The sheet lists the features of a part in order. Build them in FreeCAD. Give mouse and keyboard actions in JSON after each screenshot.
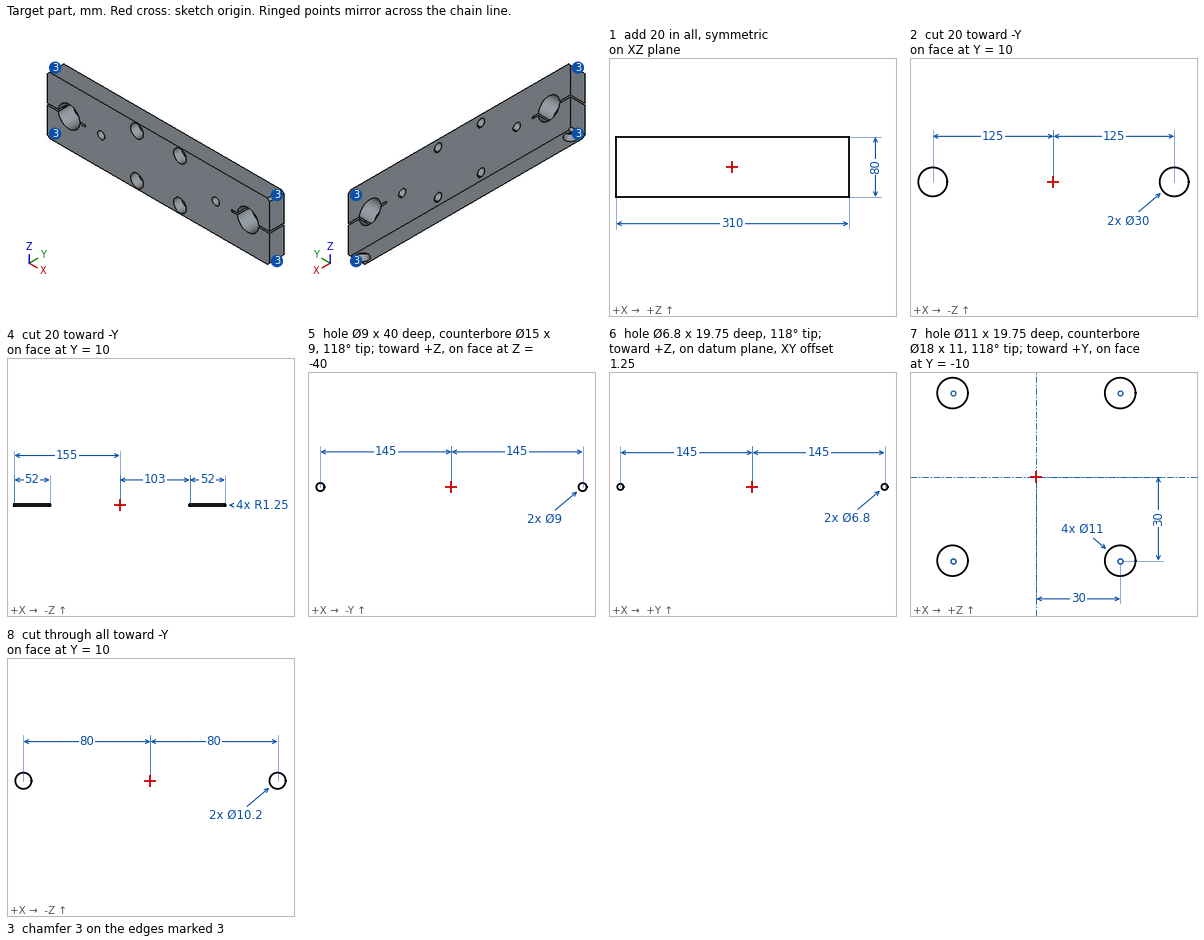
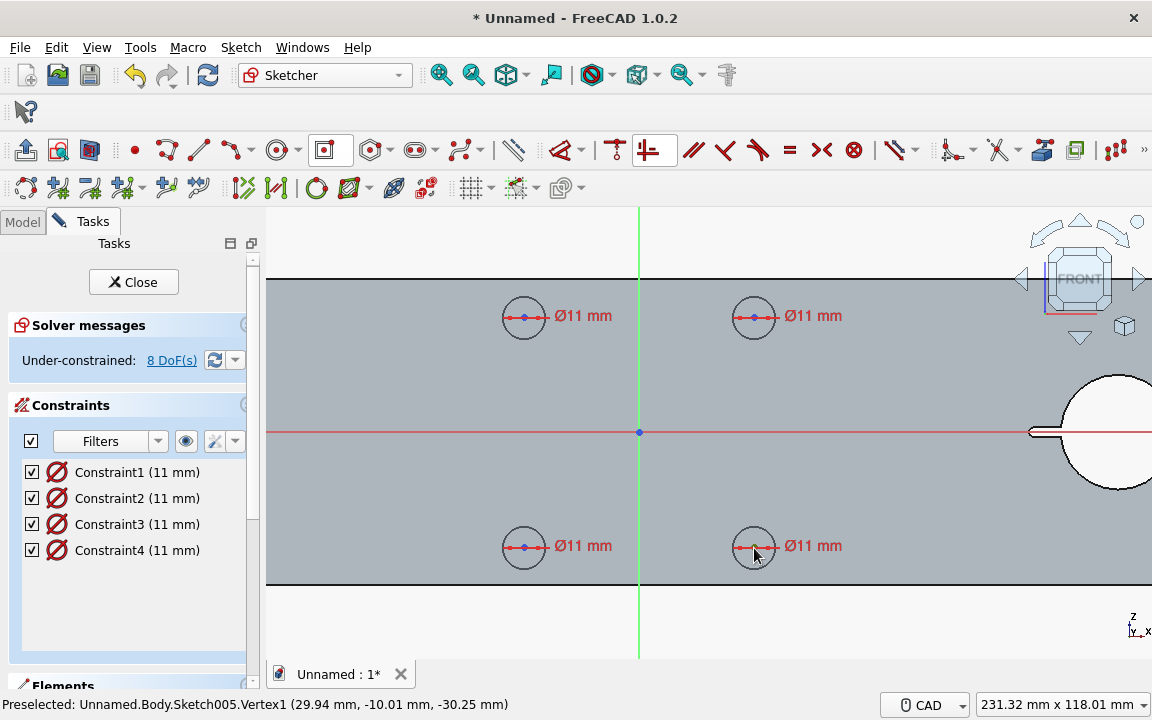
{"action": "left_click", "coordinate": [524, 548]}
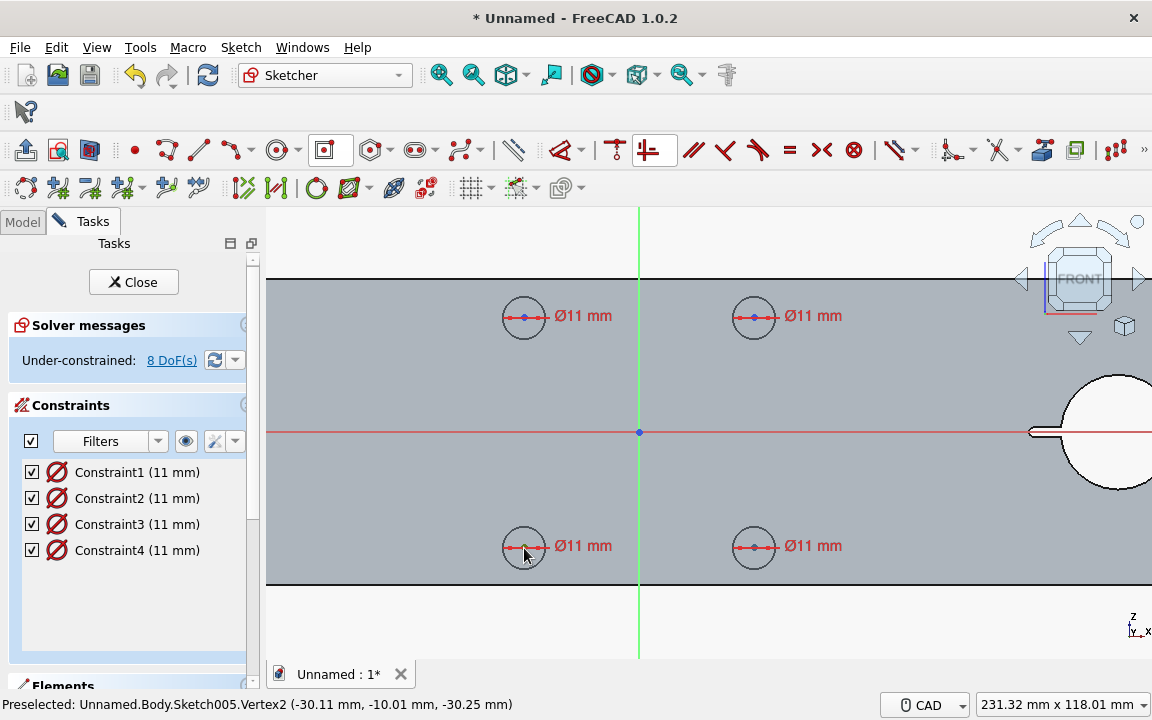
{"action": "left_click", "coordinate": [639, 603]}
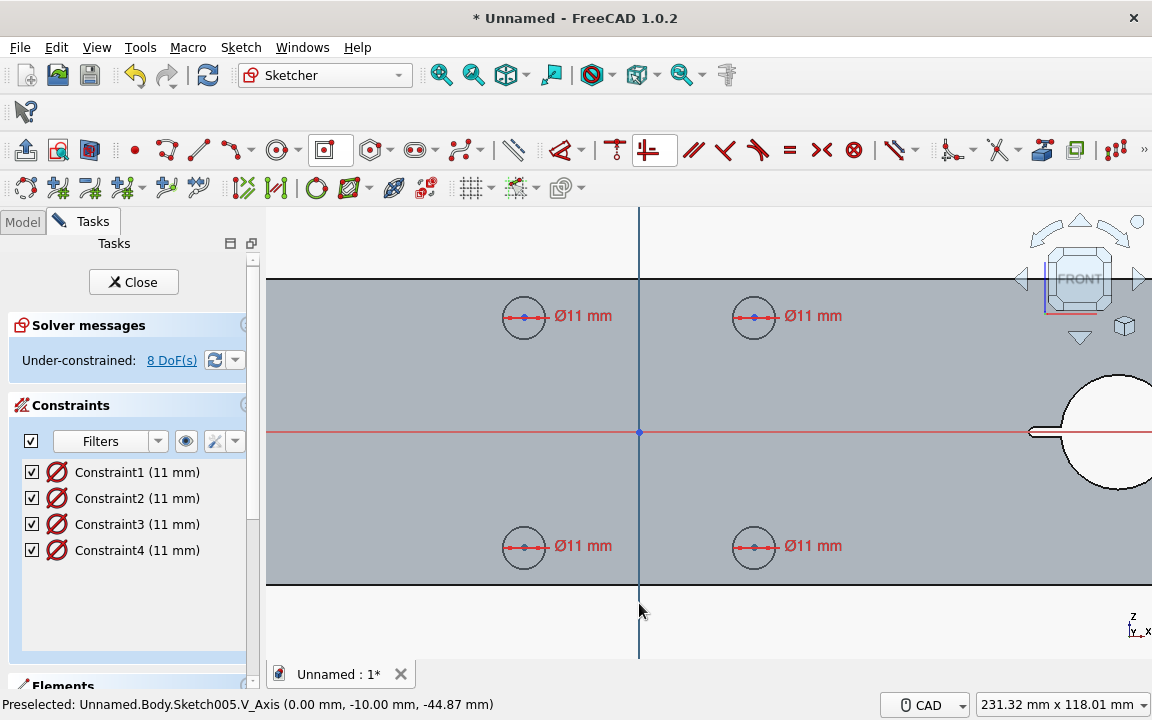
{"action": "left_click", "coordinate": [822, 150]}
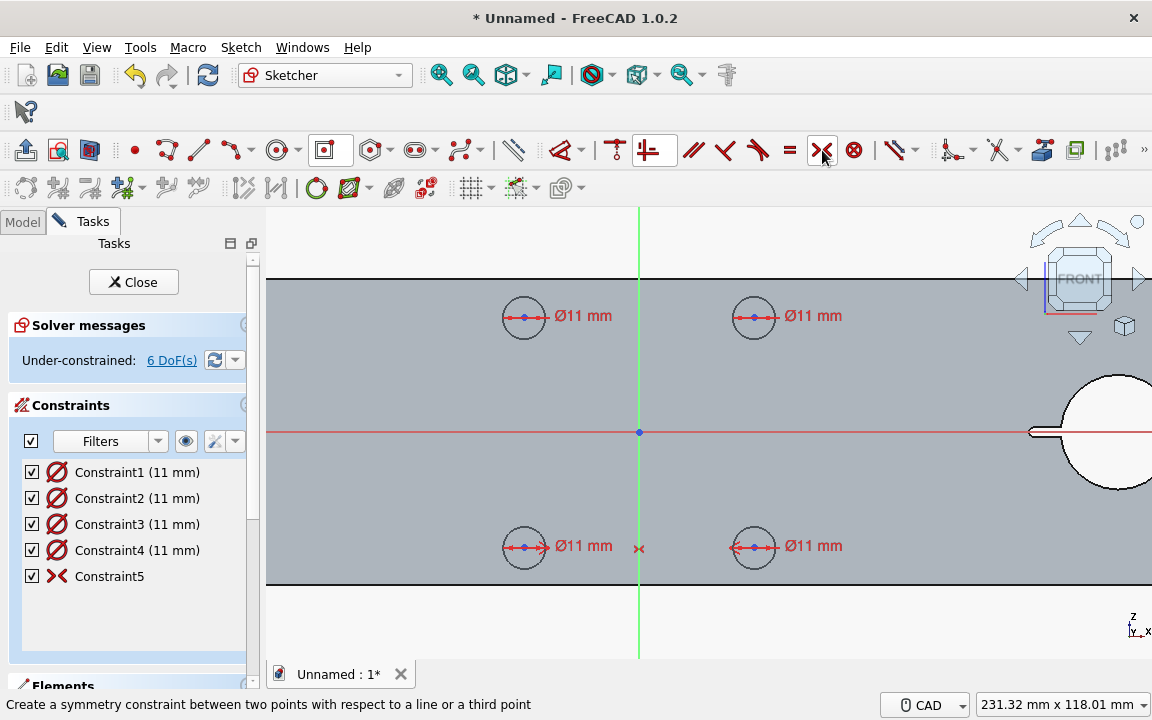
{"action": "left_click", "coordinate": [524, 548]}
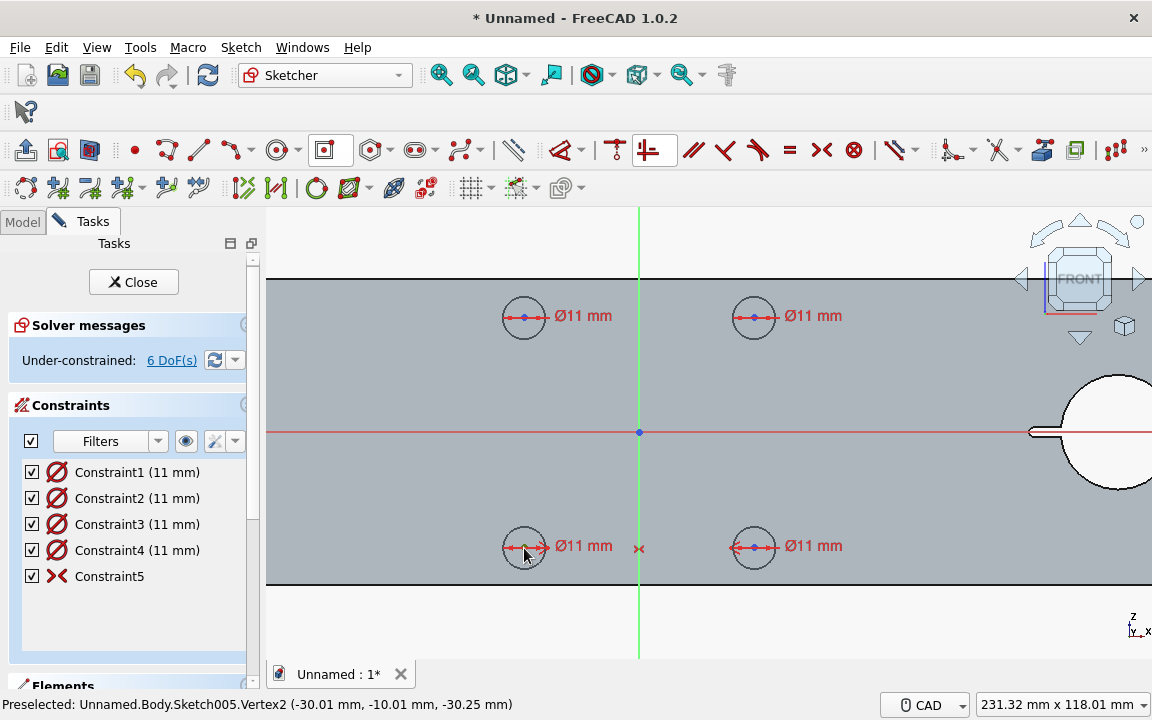
{"action": "left_click", "coordinate": [524, 318]}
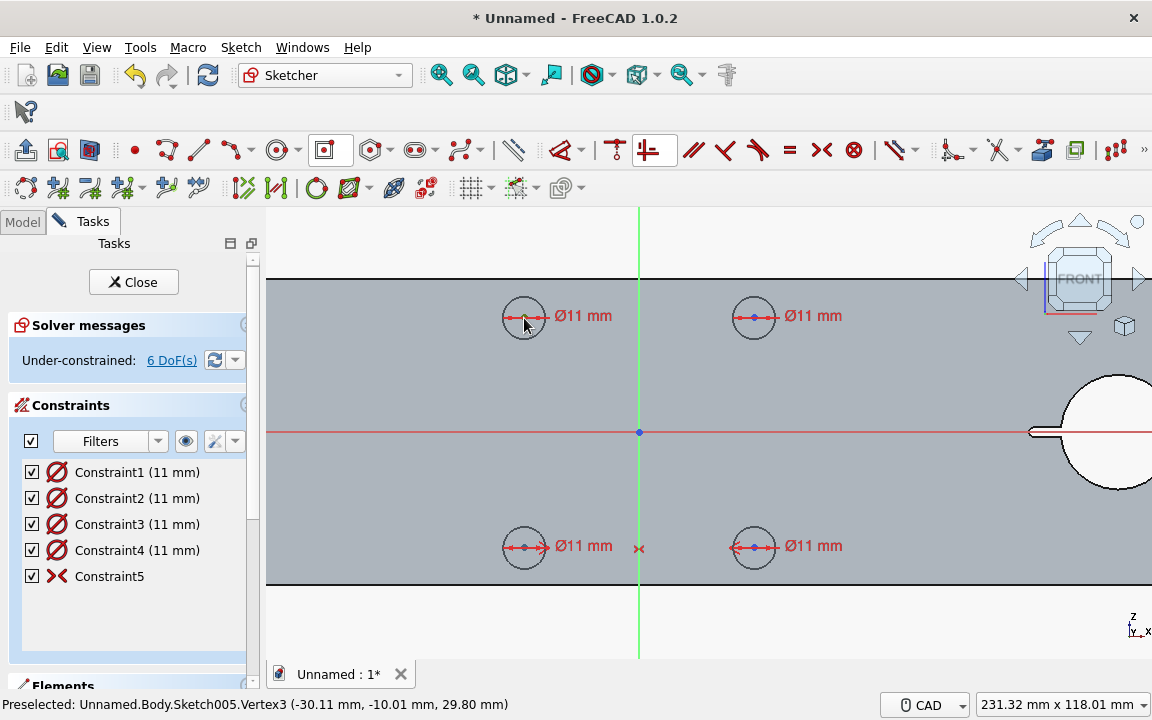
{"action": "left_click", "coordinate": [343, 432]}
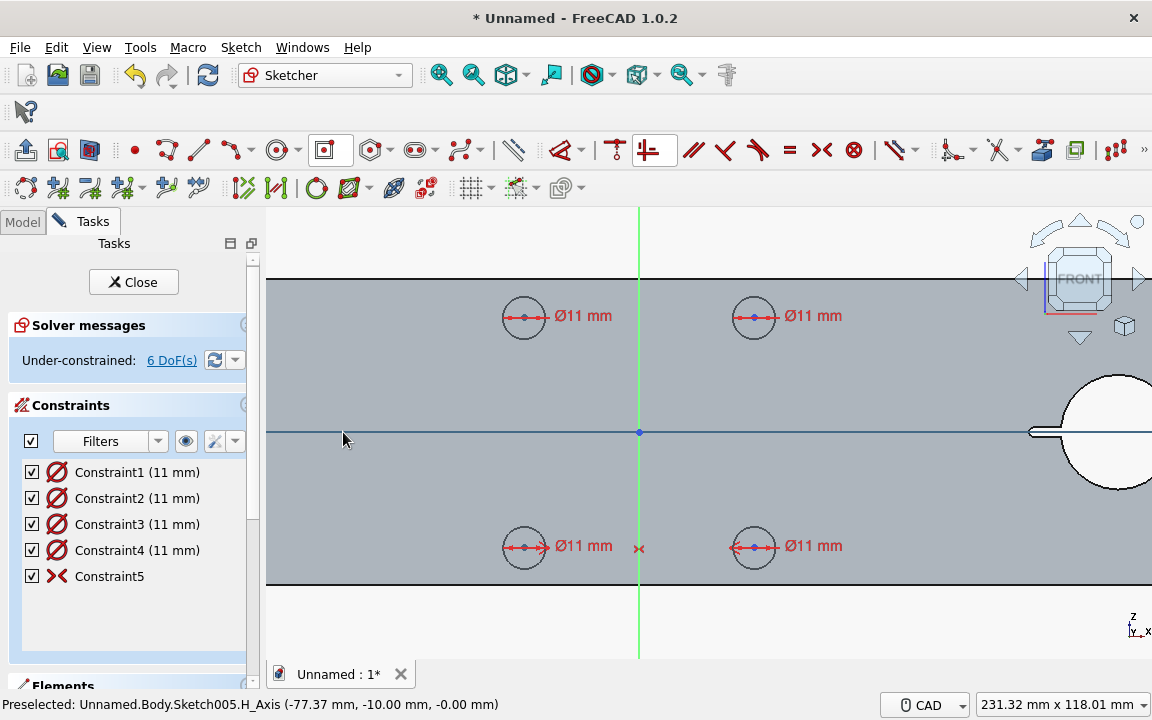
{"action": "left_click", "coordinate": [822, 150]}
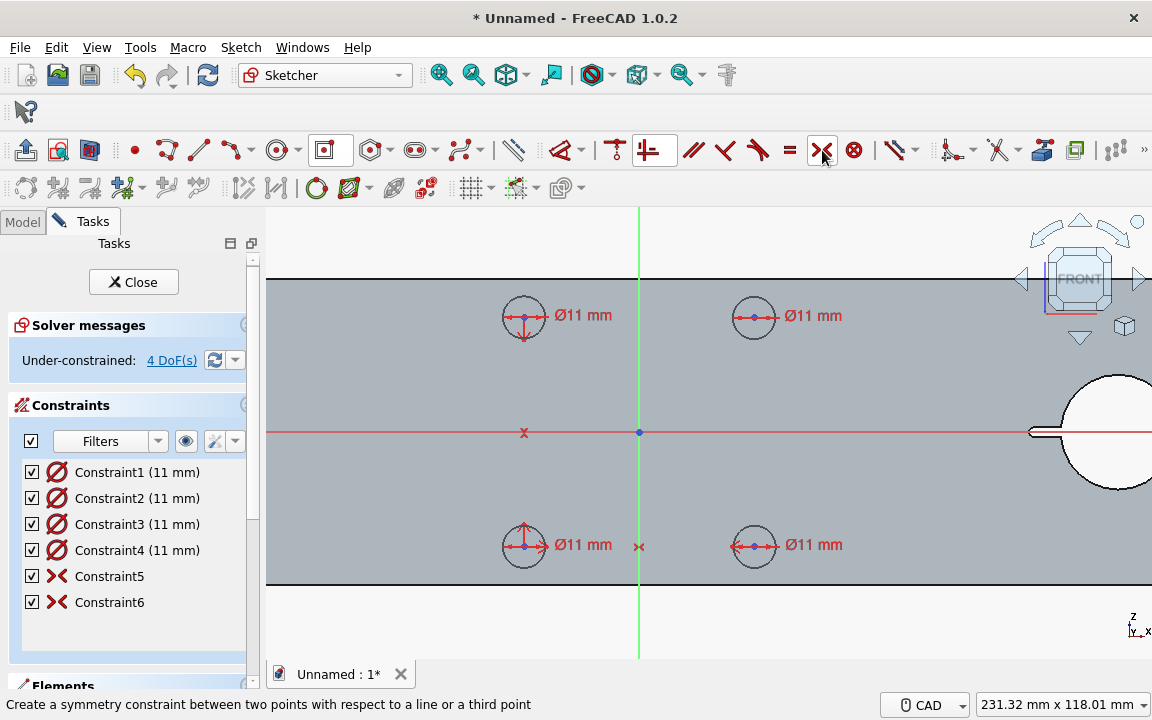
{"action": "left_click", "coordinate": [755, 547]}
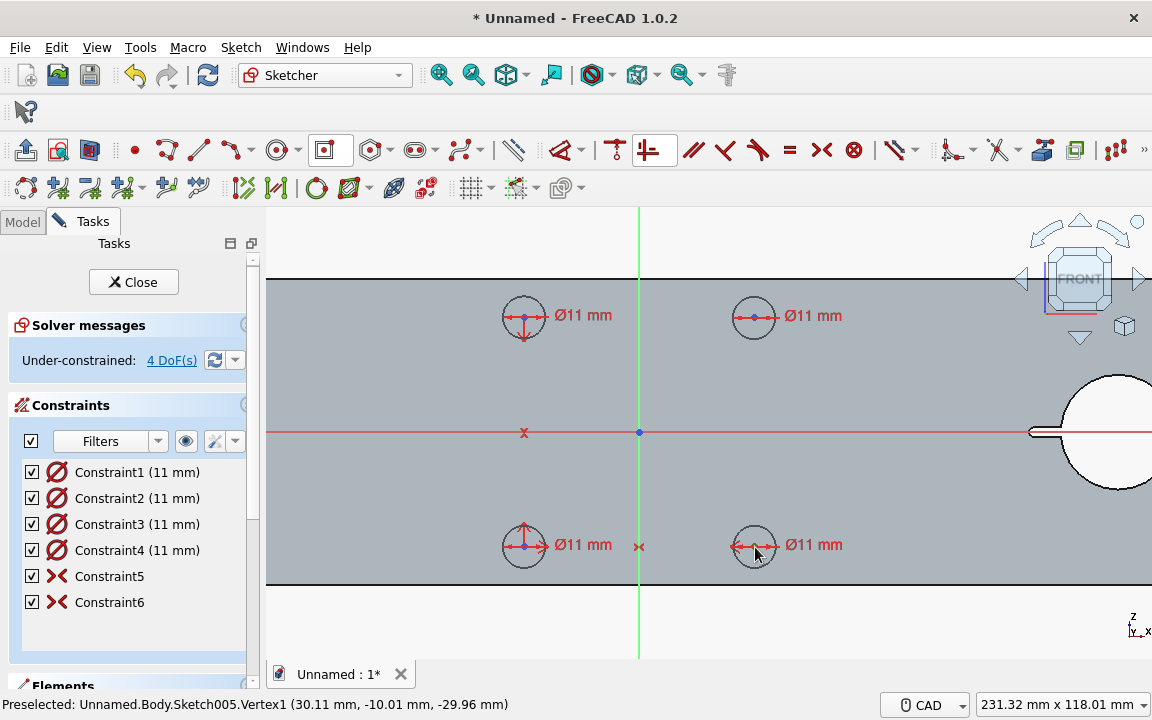
{"action": "left_click", "coordinate": [754, 318]}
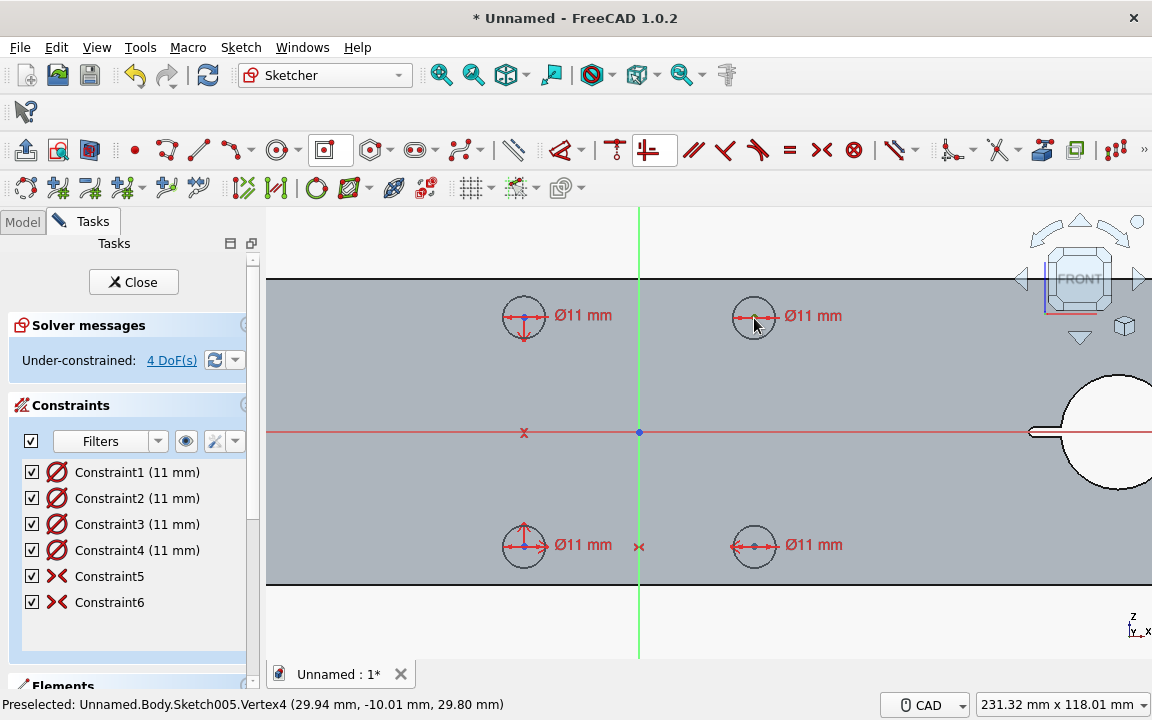
{"action": "left_click", "coordinate": [343, 432]}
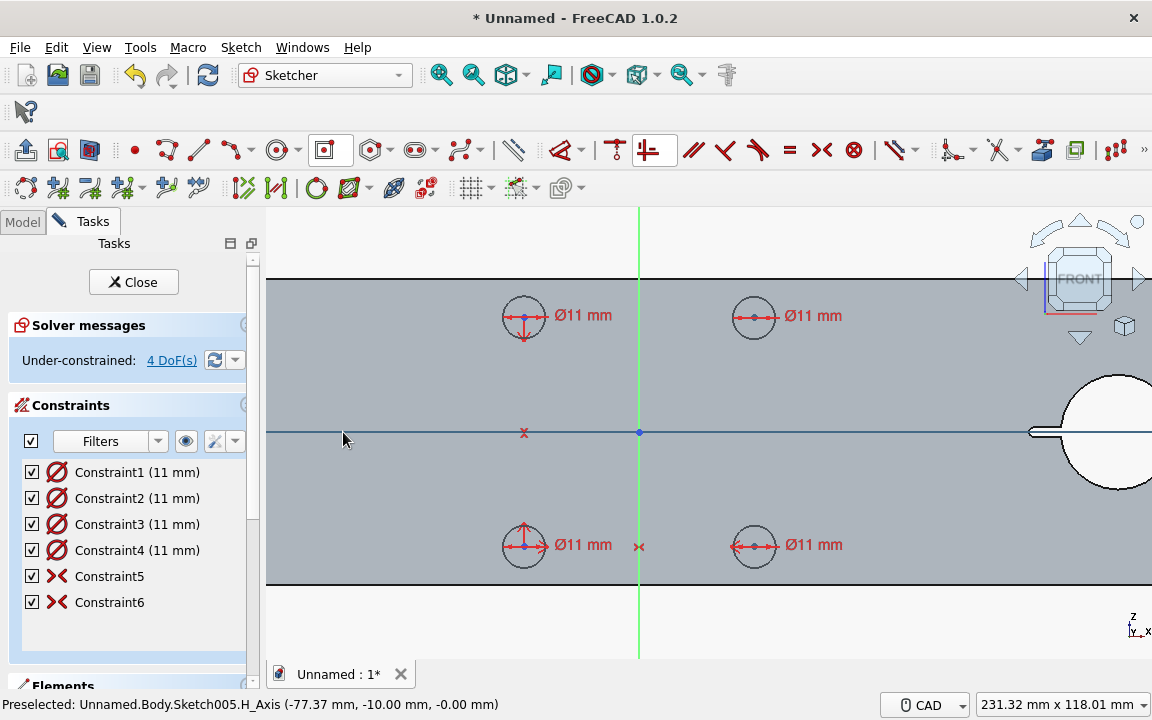
{"action": "left_click", "coordinate": [822, 150]}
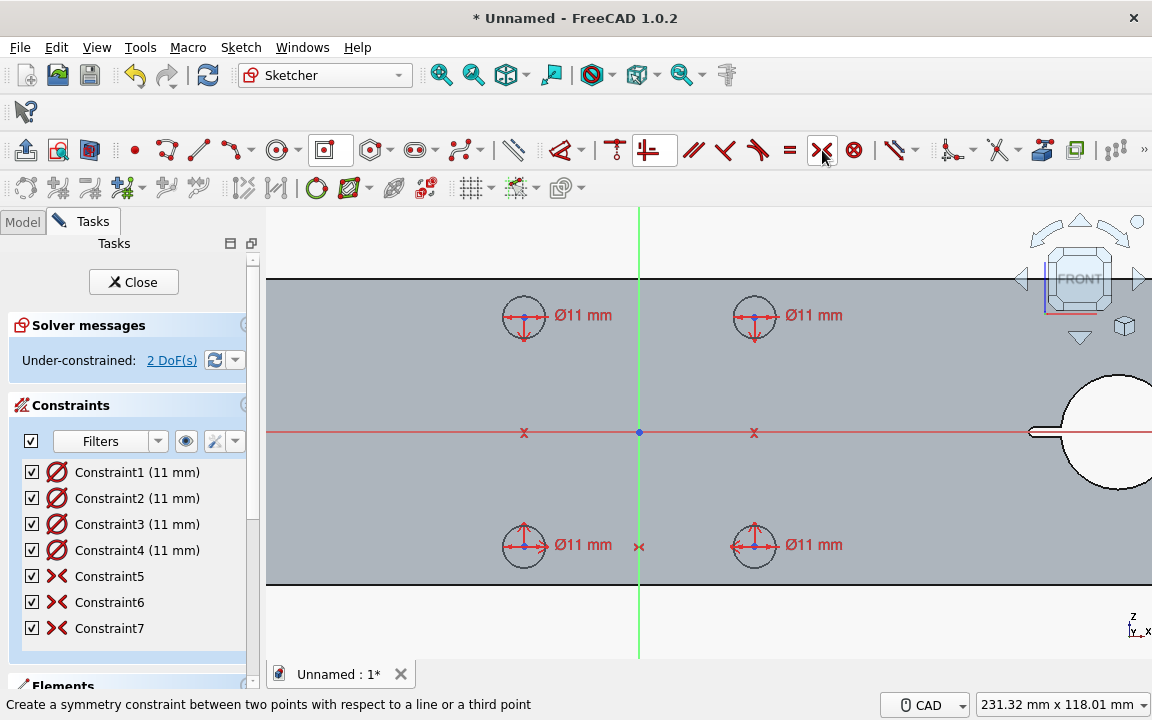
{"action": "left_click", "coordinate": [560, 150]}